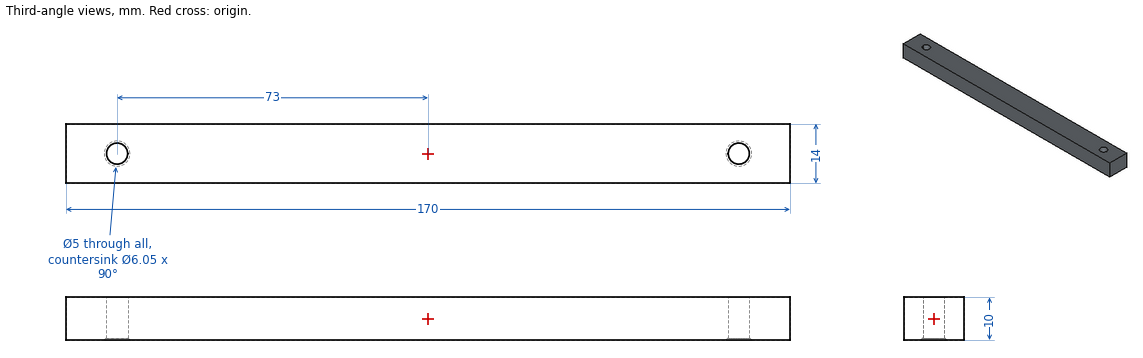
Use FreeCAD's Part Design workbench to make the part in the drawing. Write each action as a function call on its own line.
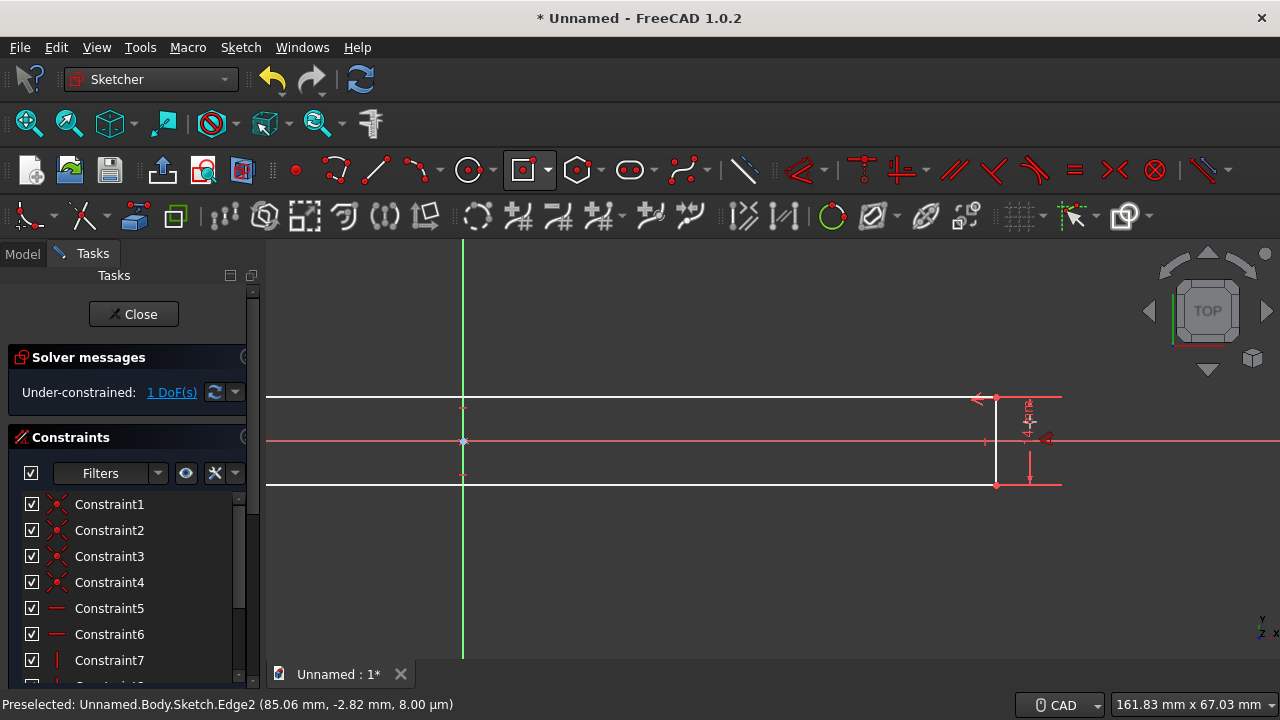
click(677, 485)
click(645, 519)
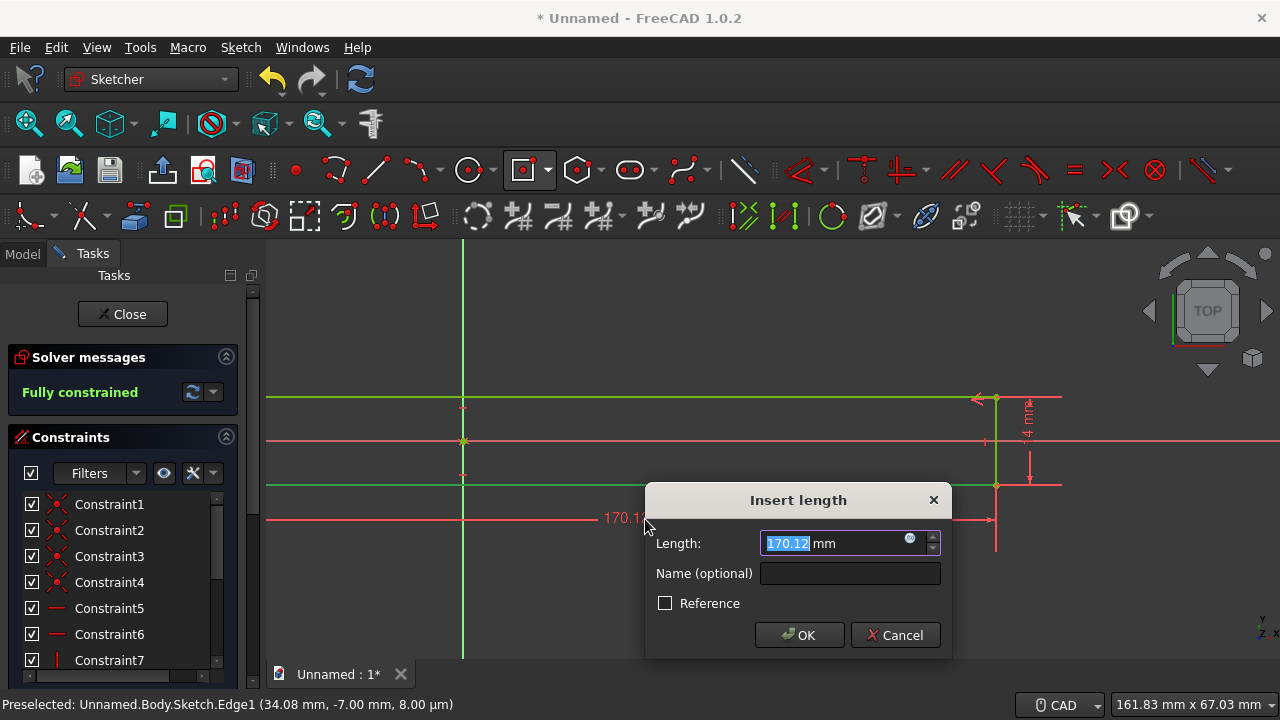
text(170)
key(Return)
key(Escape)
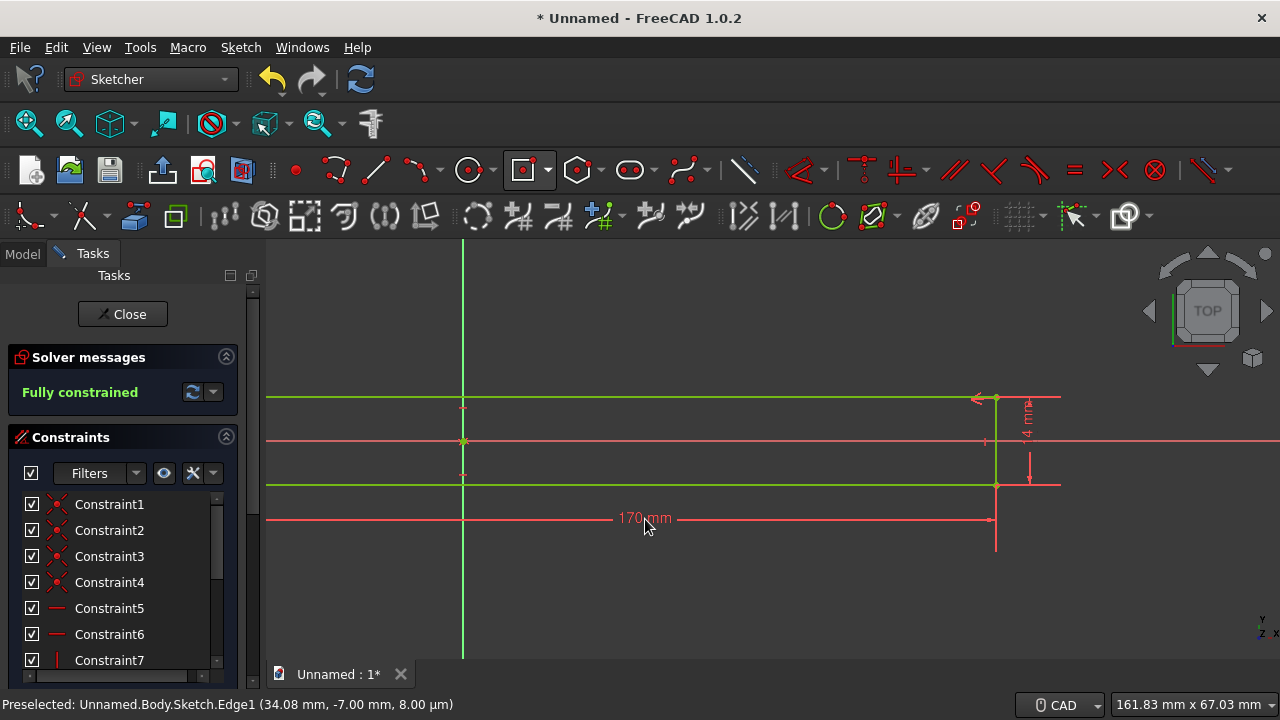
click(123, 314)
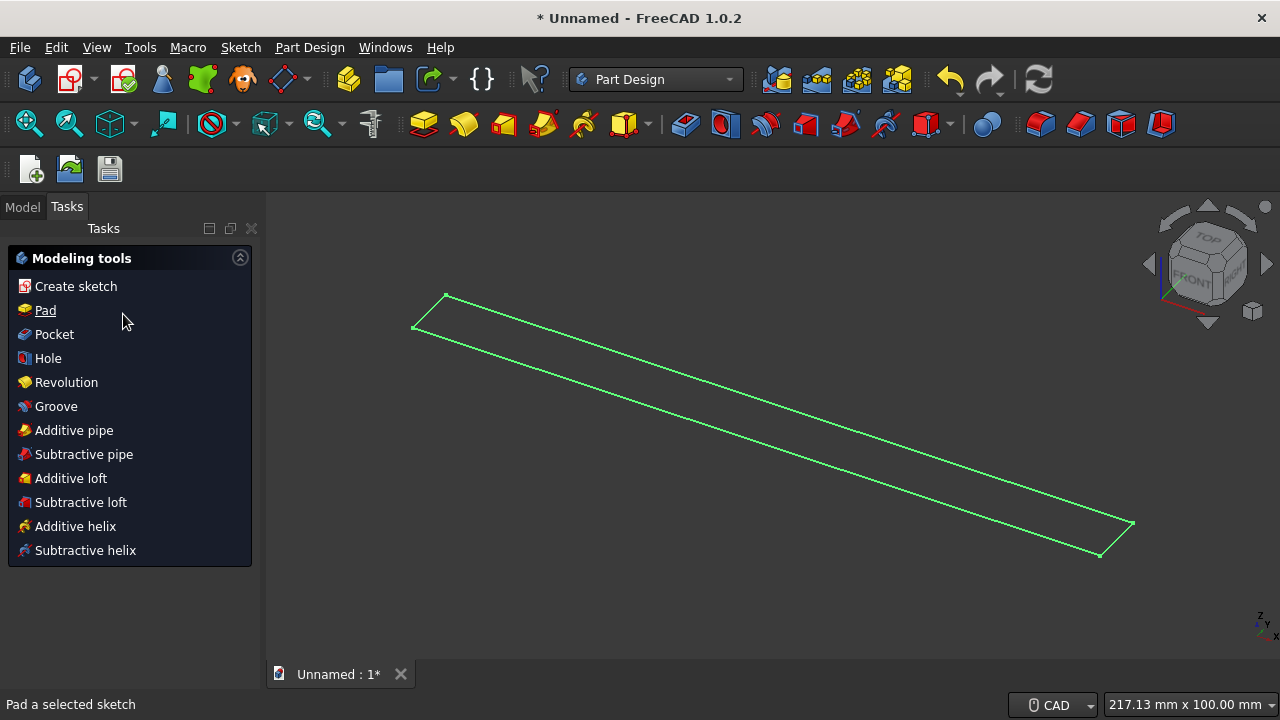
click(424, 124)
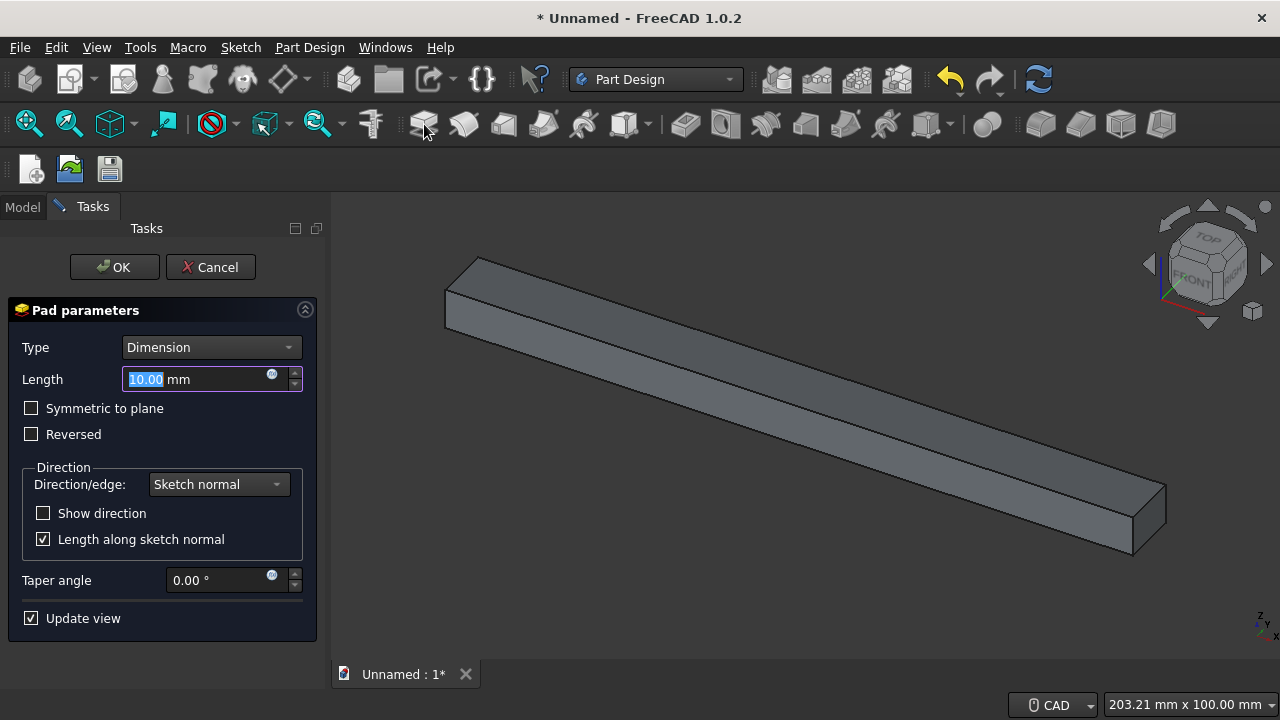
text(10)
key(Tab)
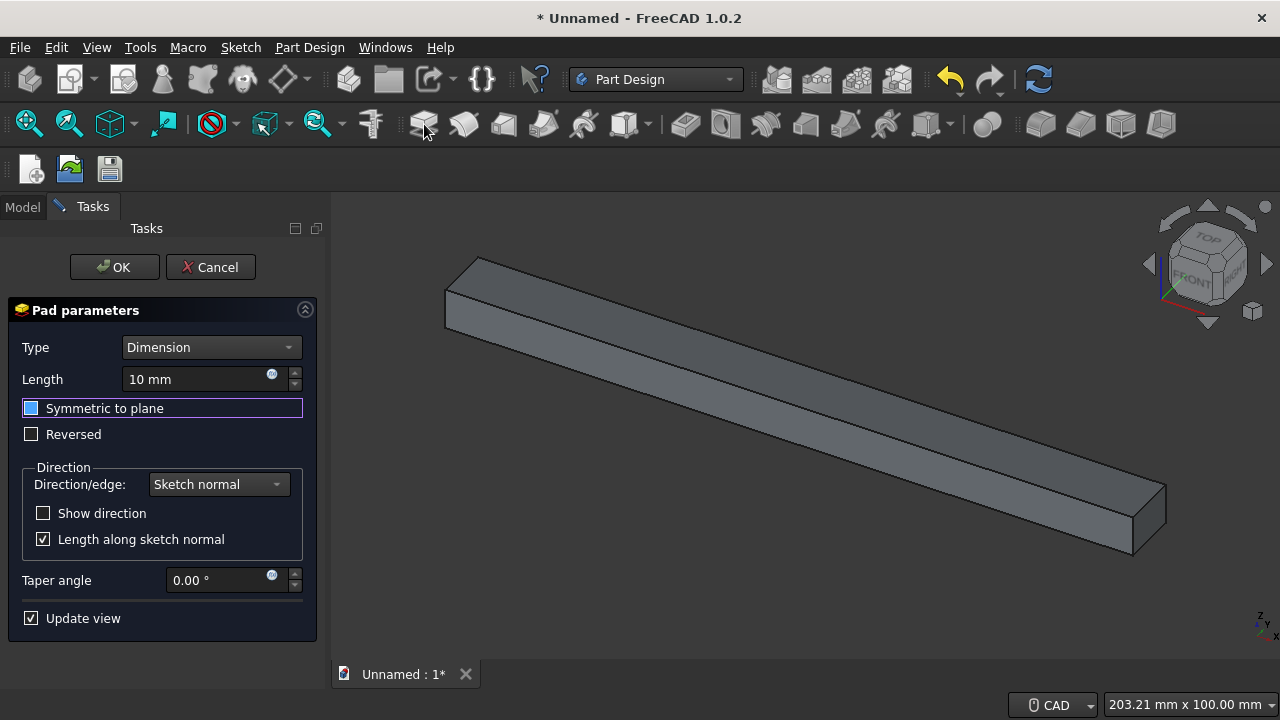
click(30, 408)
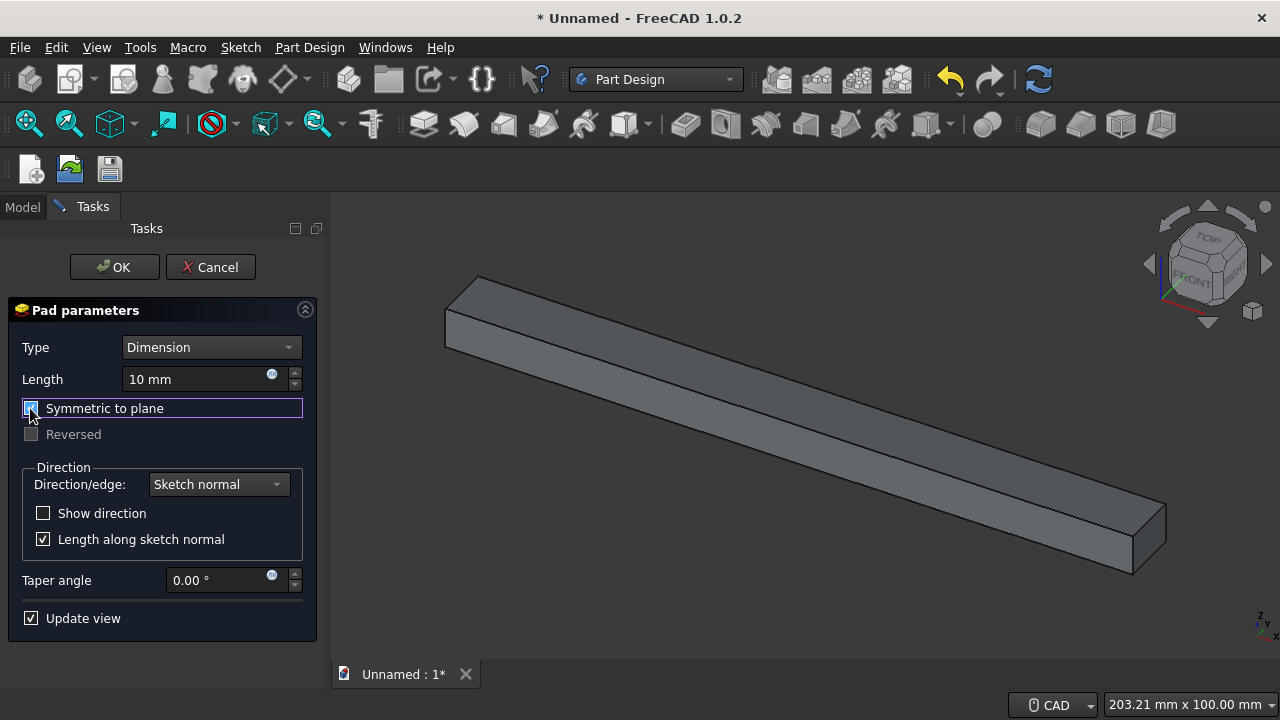
click(115, 267)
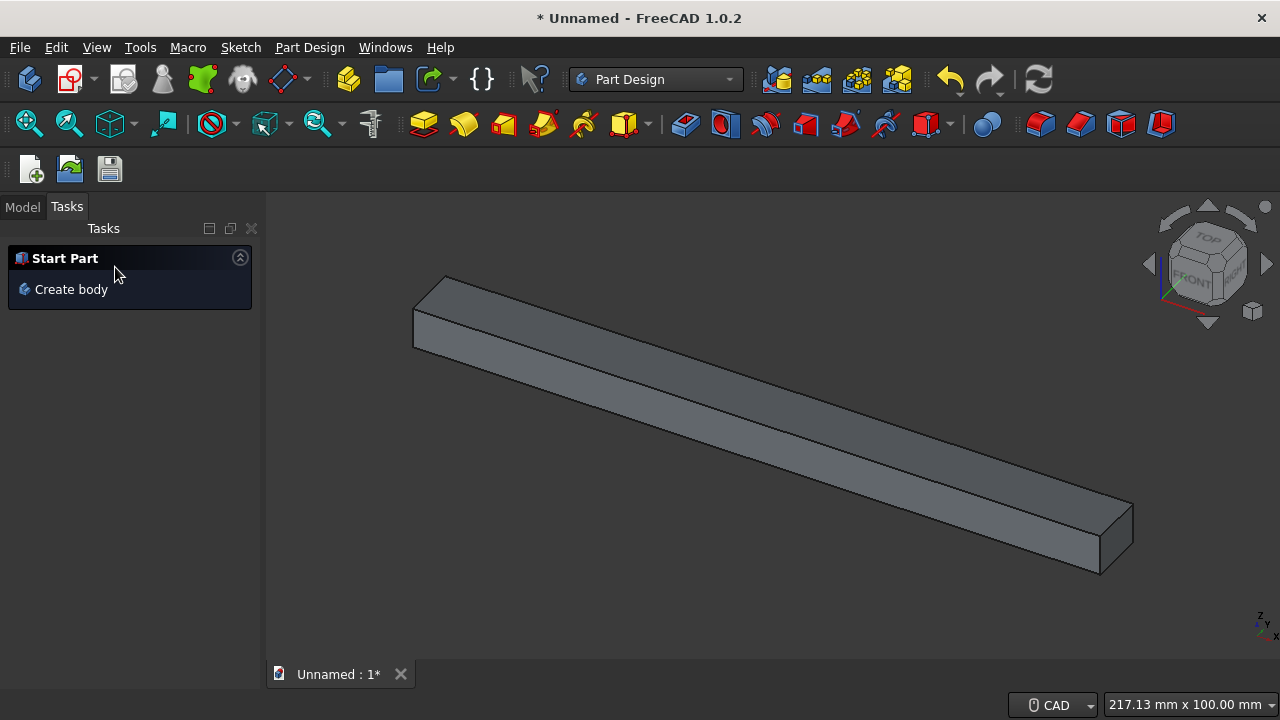
key(5)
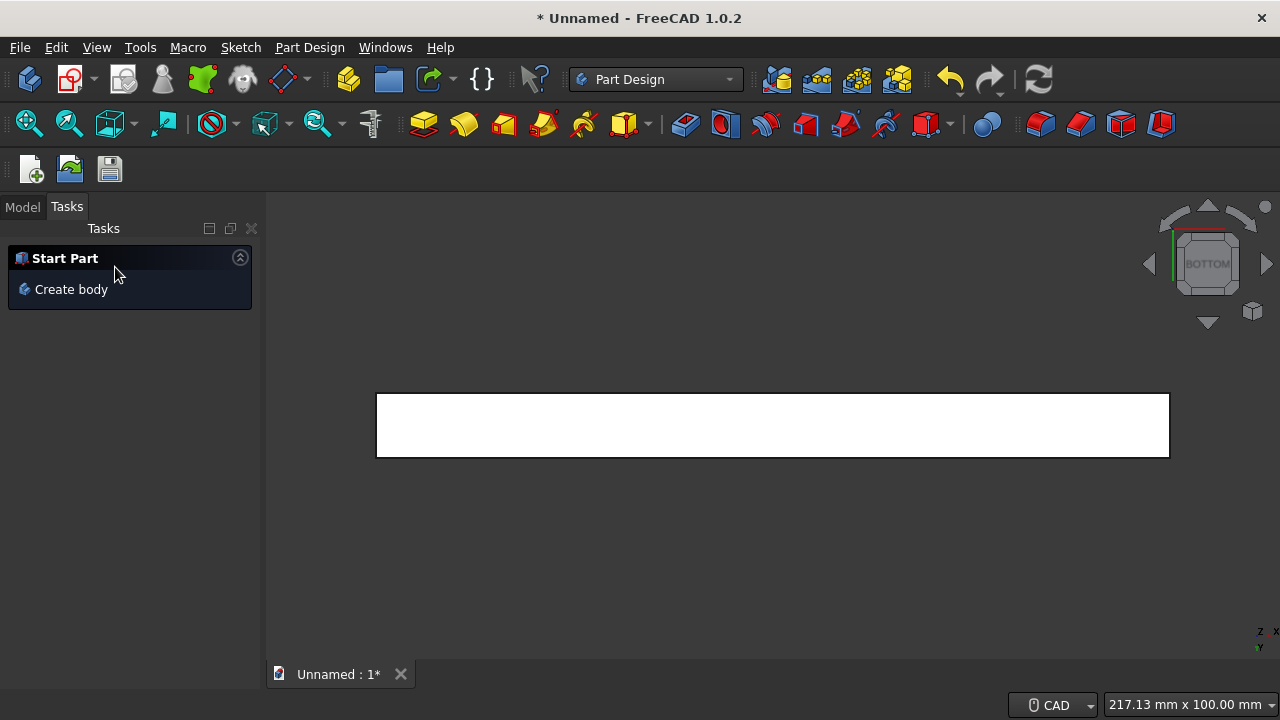
click(1113, 424)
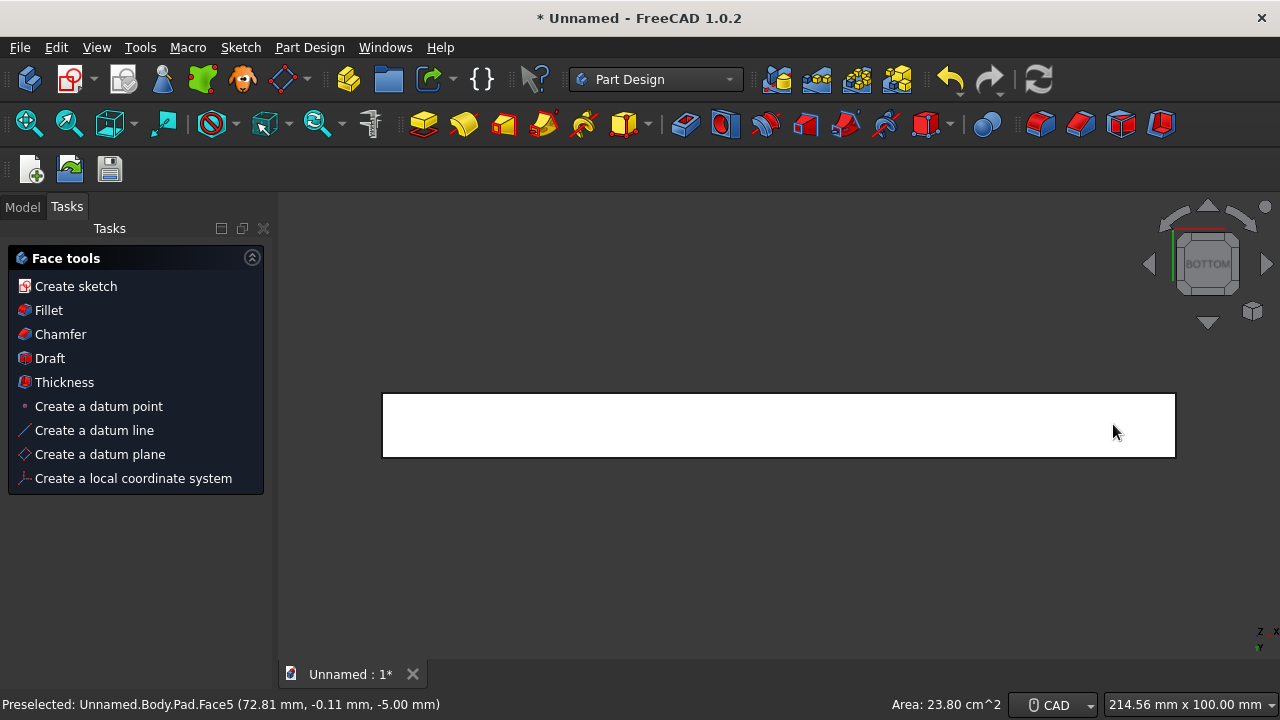
click(70, 80)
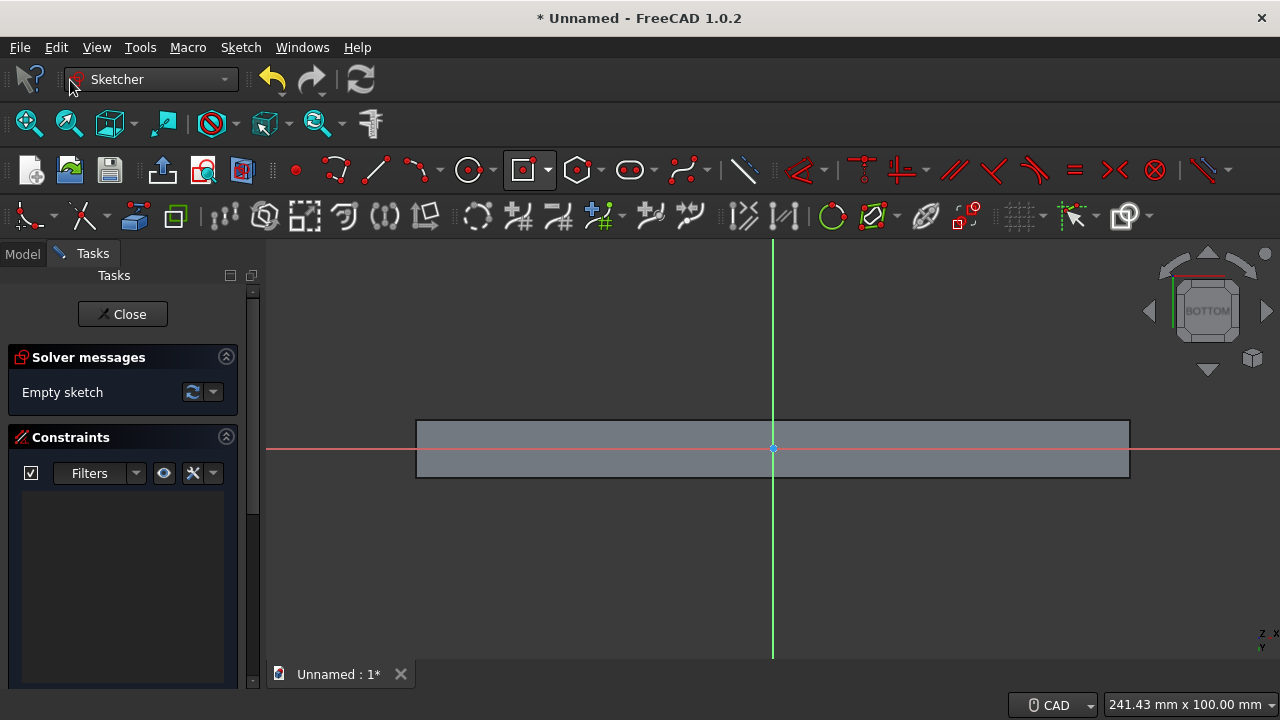
scroll(447, 449, up, 13)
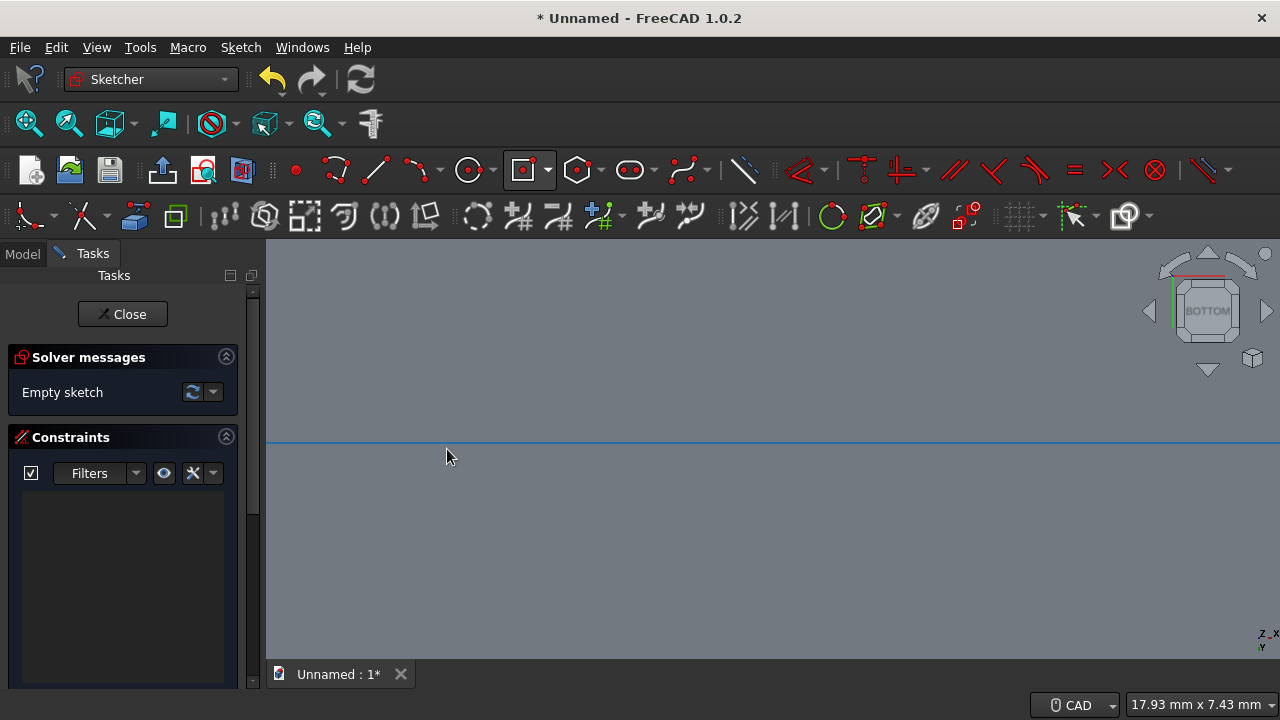
click(470, 170)